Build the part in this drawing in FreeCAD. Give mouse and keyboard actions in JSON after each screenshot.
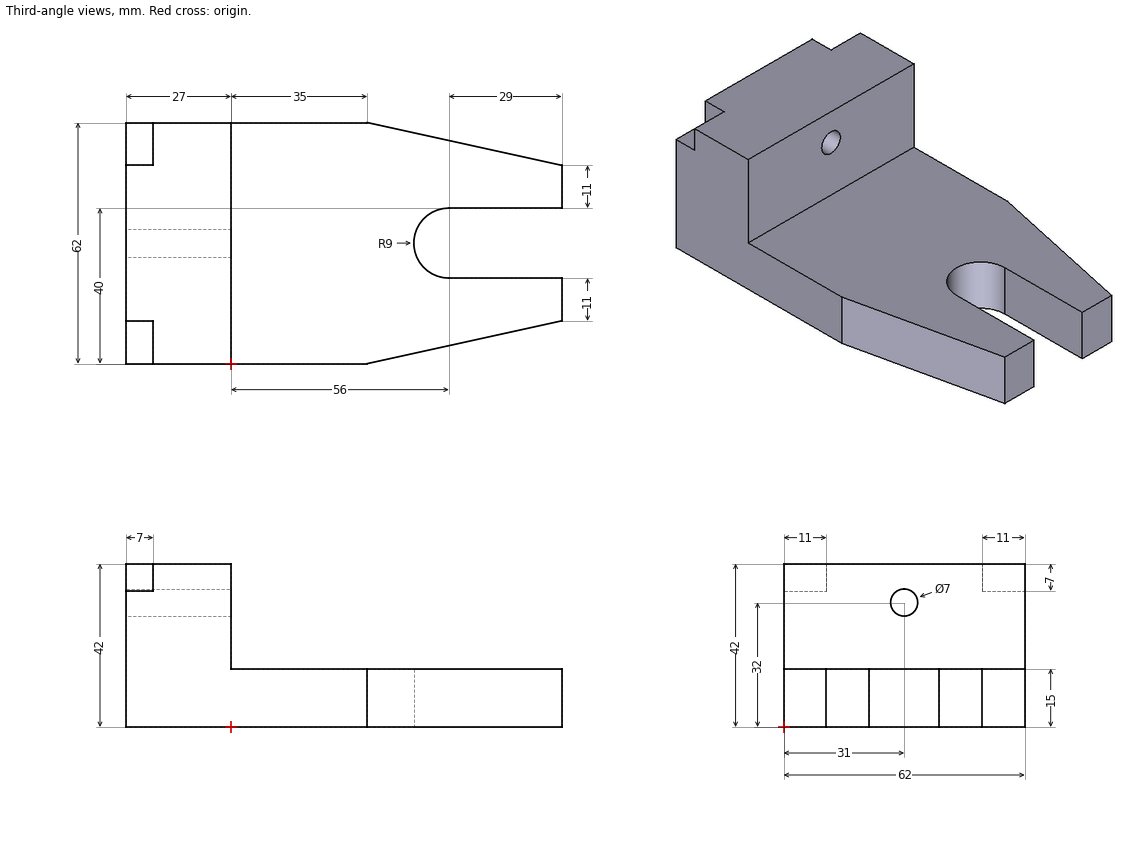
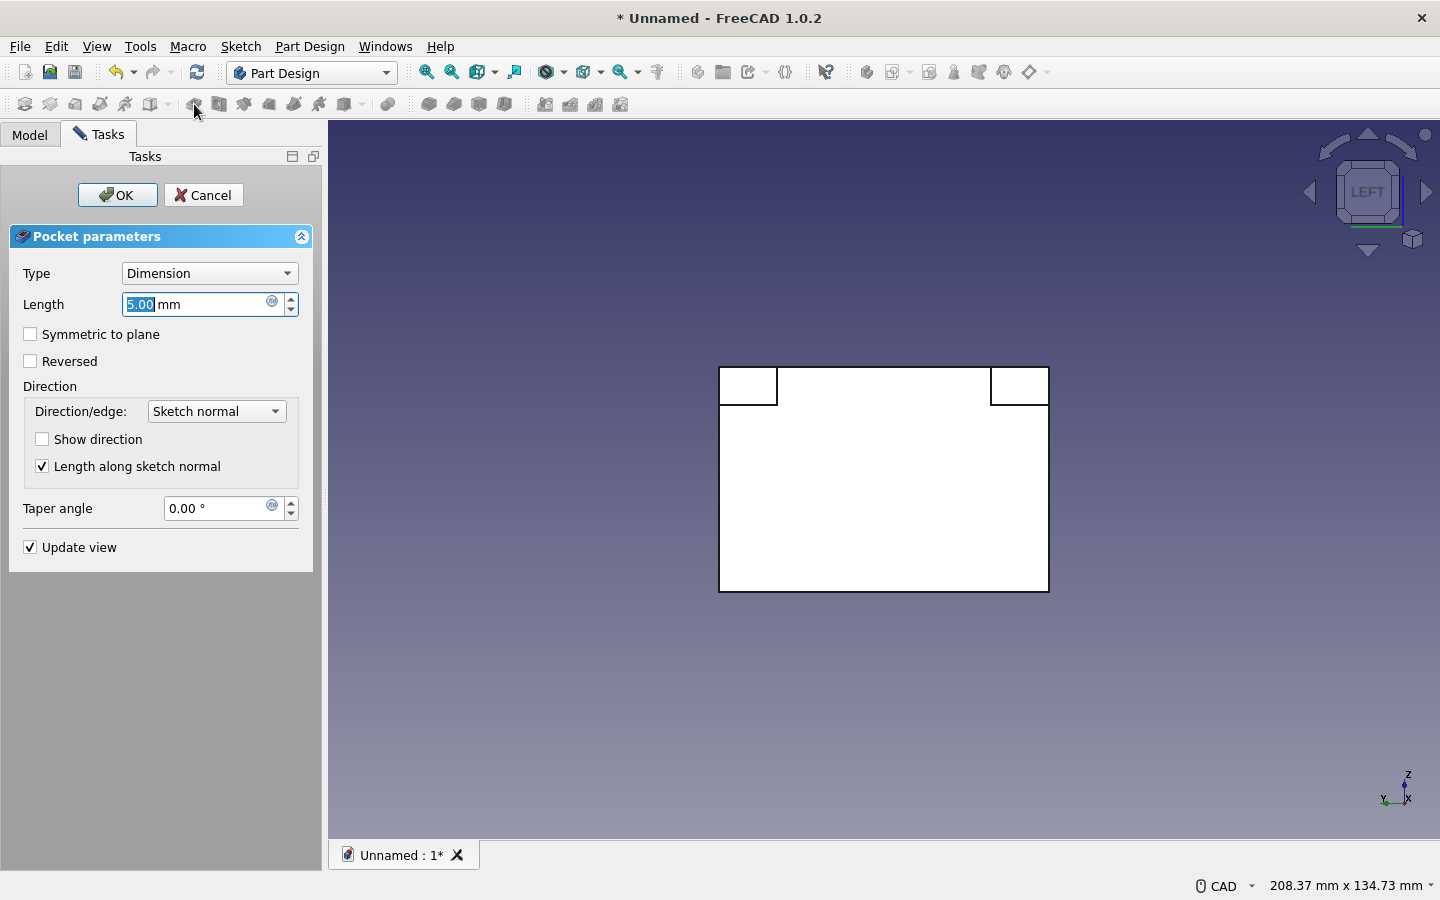
{"action": "type", "text": "7"}
{"action": "key", "text": "Tab"}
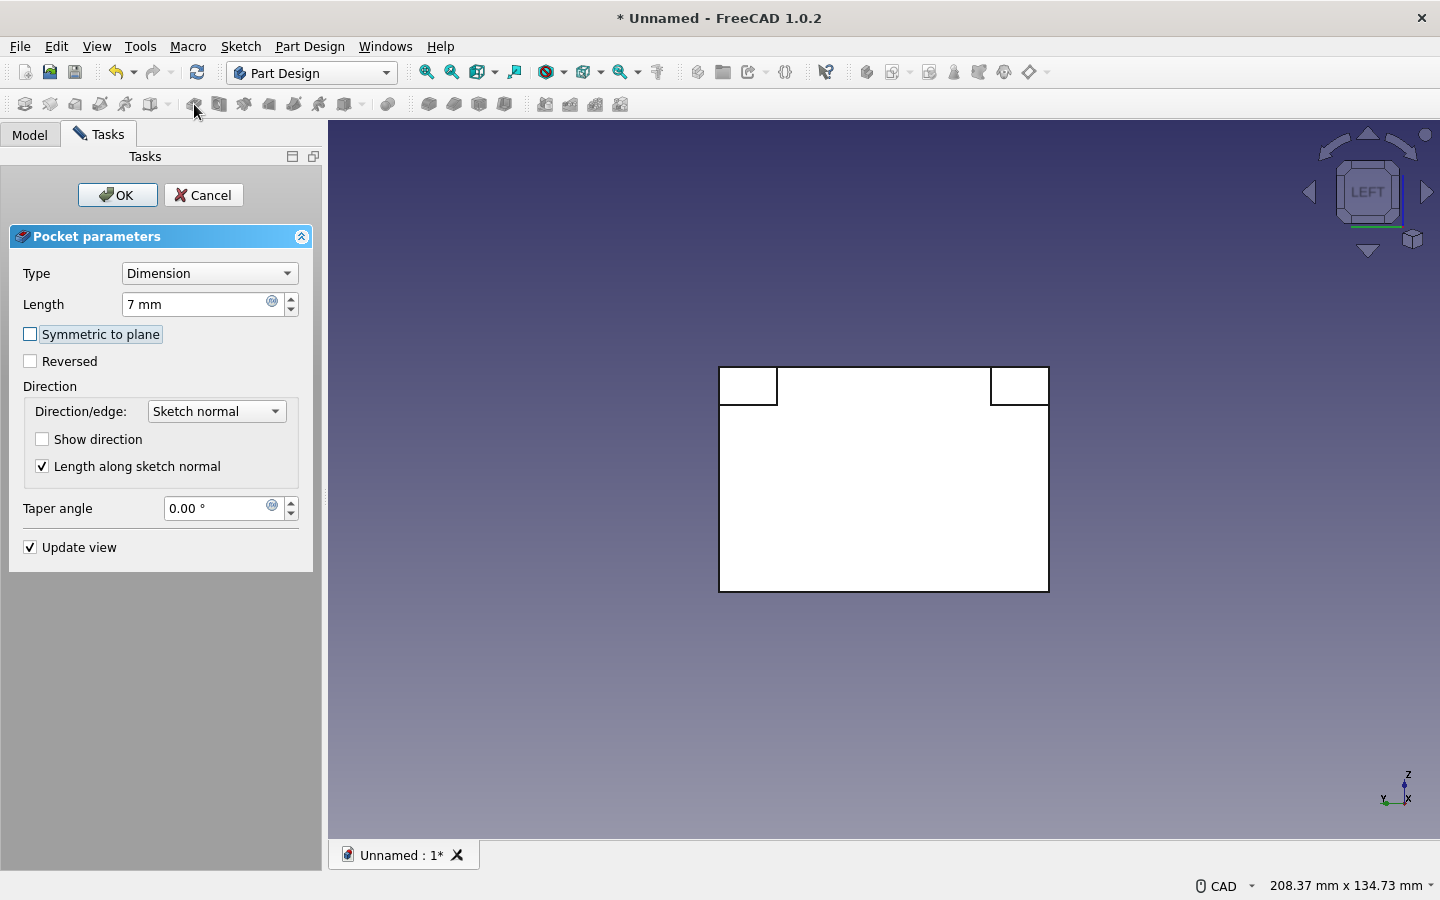
{"action": "left_click", "coordinate": [118, 195]}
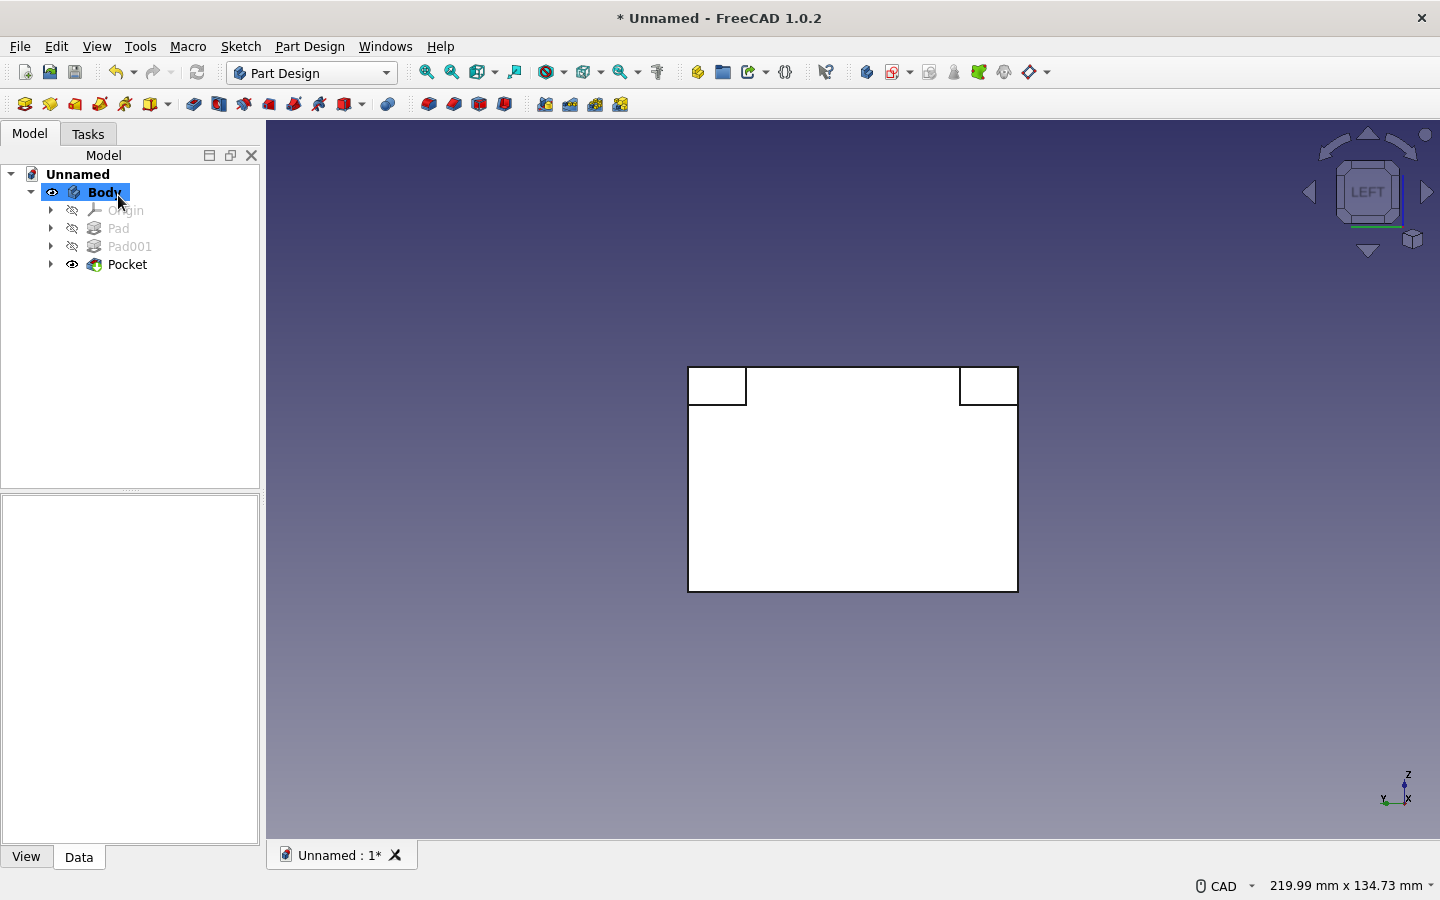
{"action": "left_click", "coordinate": [427, 72]}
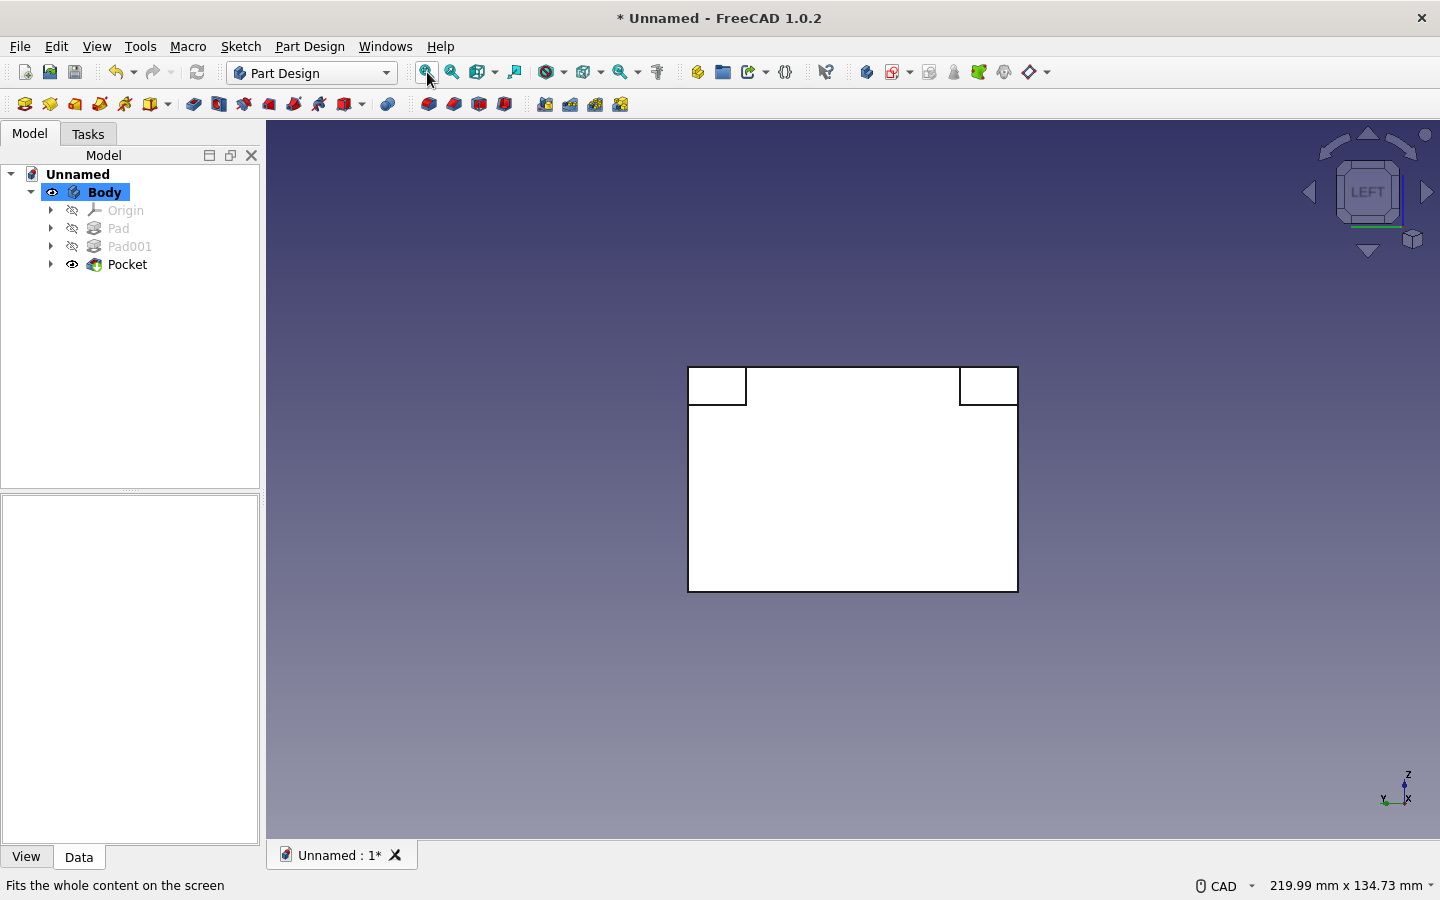
{"action": "left_click", "coordinate": [853, 478]}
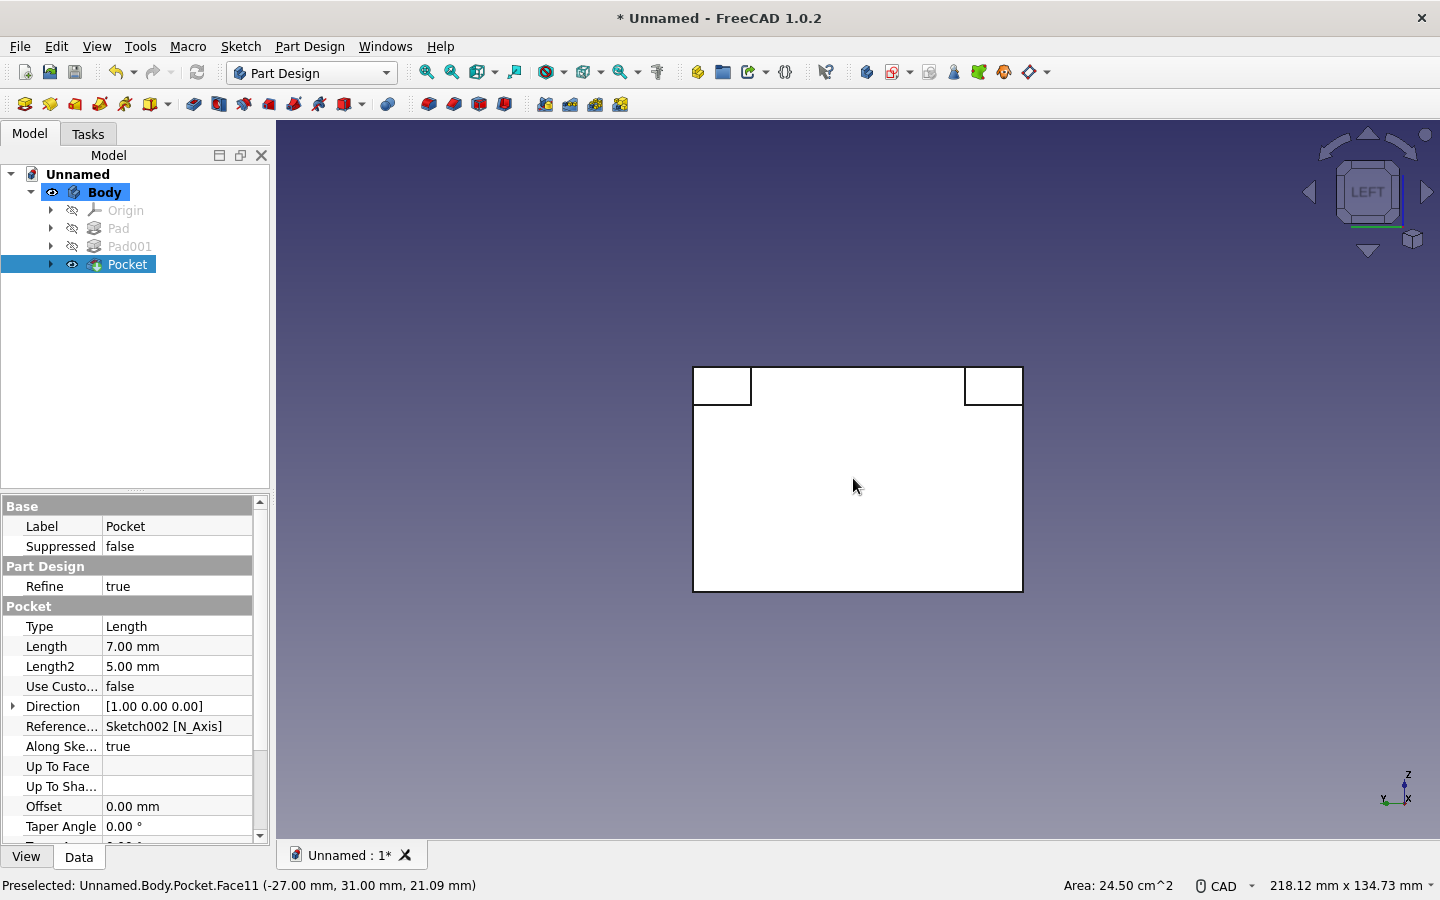
{"action": "left_click", "coordinate": [892, 72]}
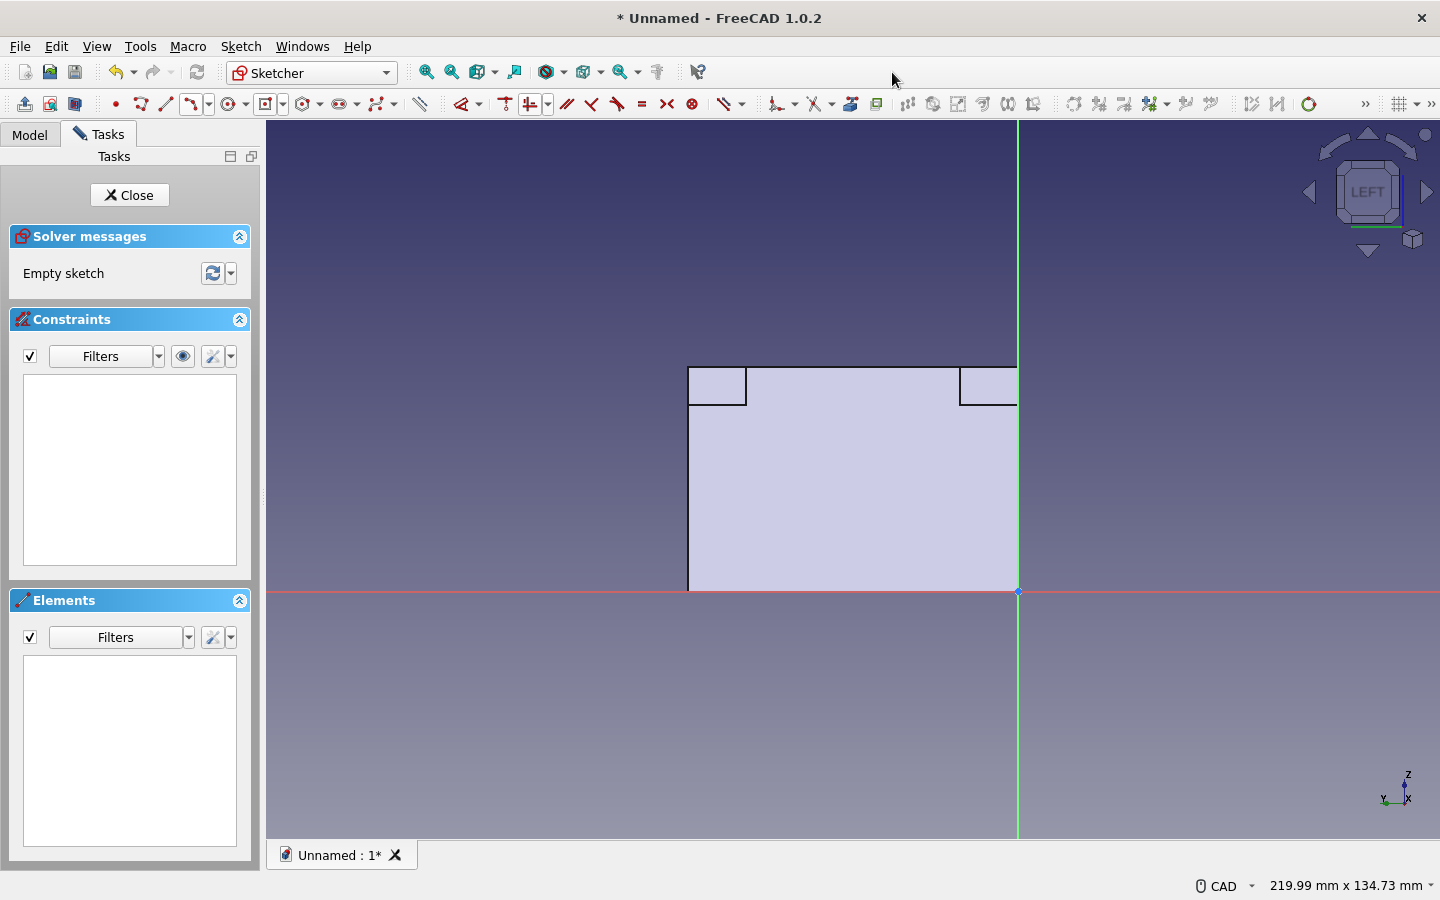
{"action": "scroll", "coordinate": [858, 416], "scroll_direction": "up", "scroll_amount": 13}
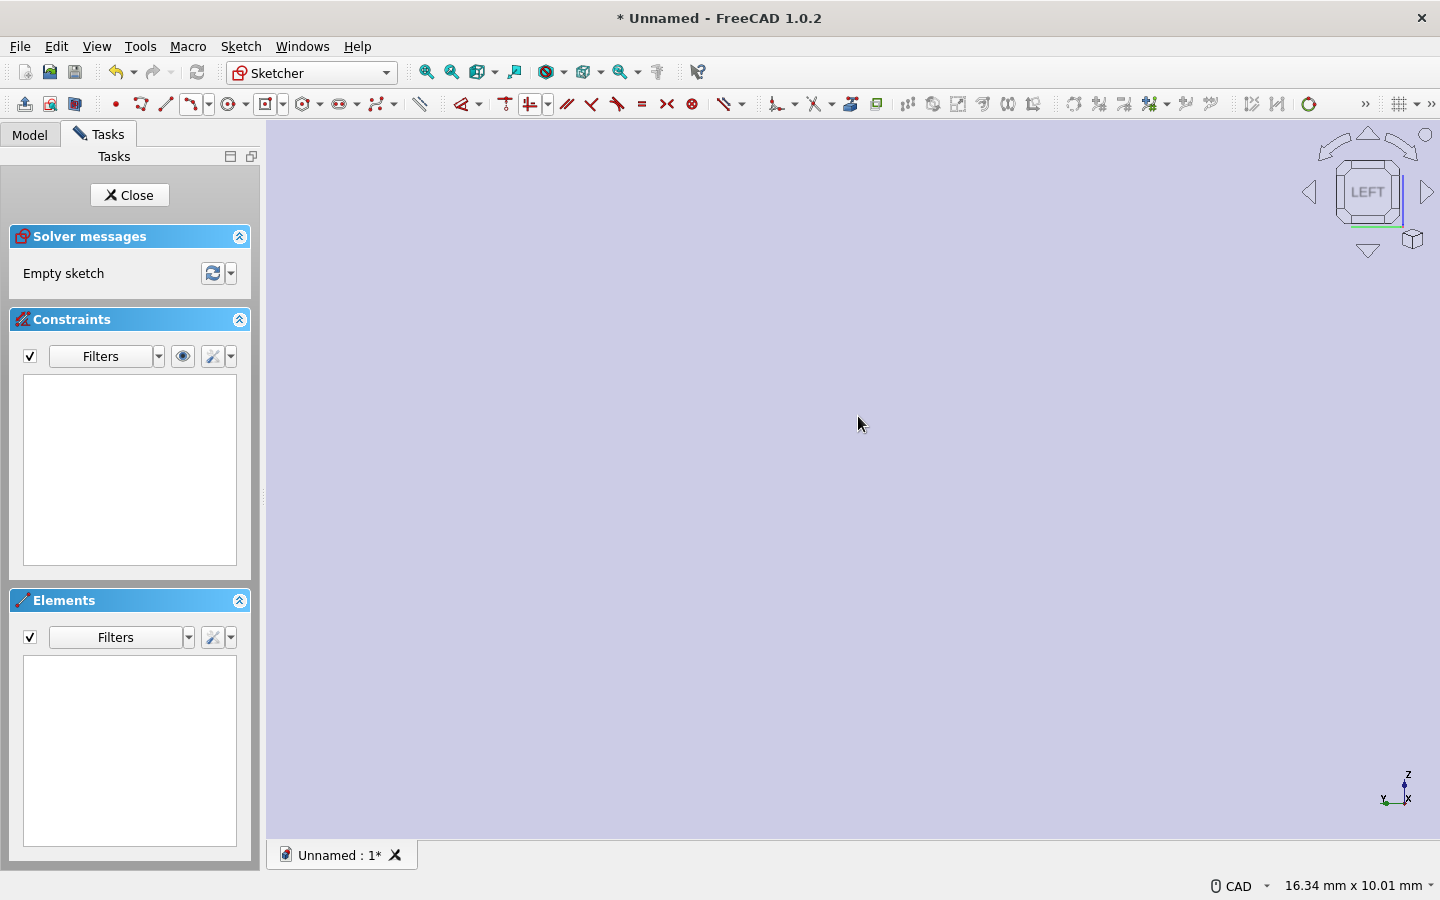
{"action": "left_click", "coordinate": [228, 104]}